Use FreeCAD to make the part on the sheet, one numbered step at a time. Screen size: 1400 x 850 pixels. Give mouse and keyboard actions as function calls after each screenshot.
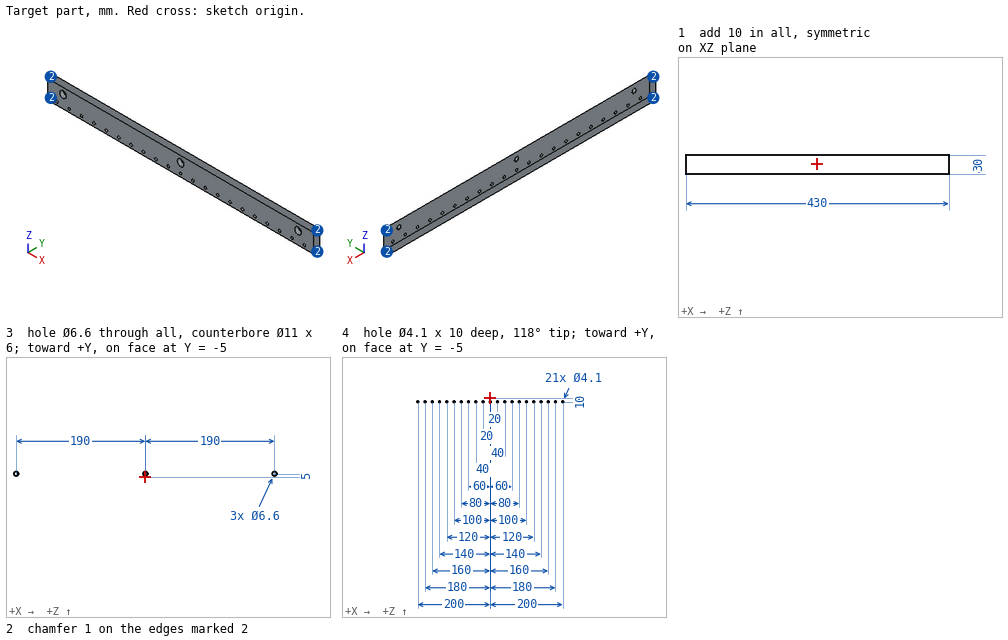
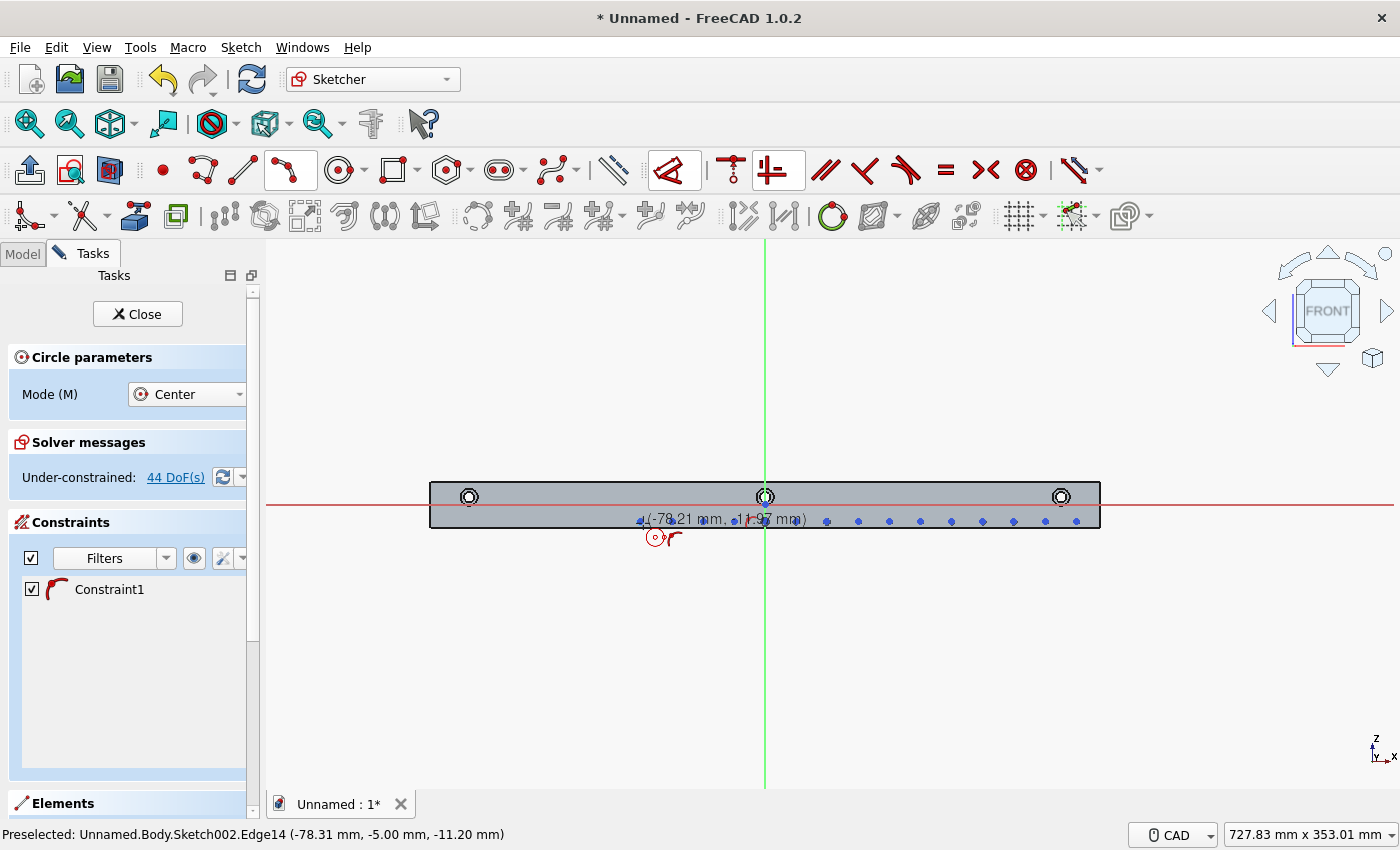
click(609, 521)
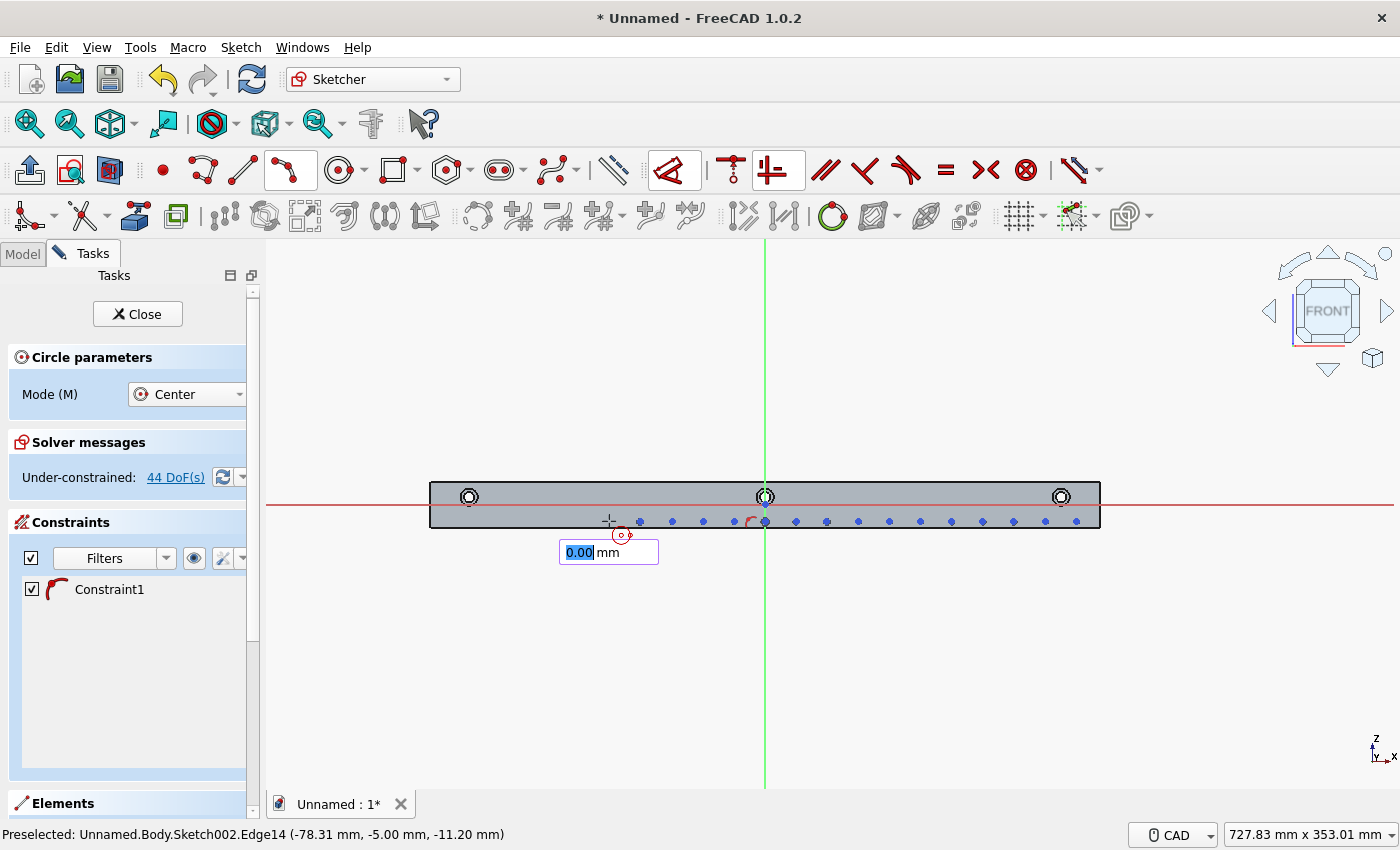
scroll(612, 523, up, 9)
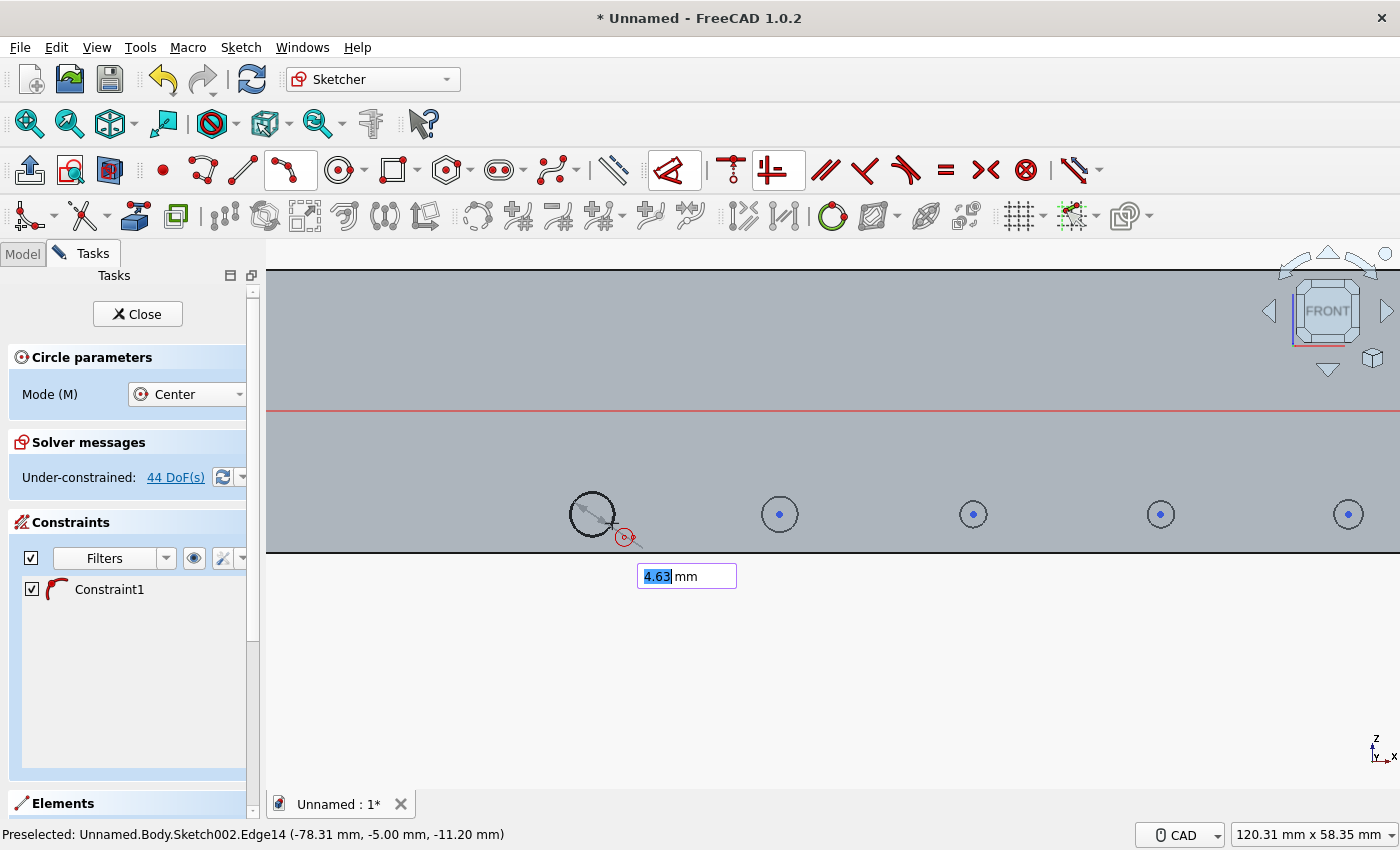
click(608, 519)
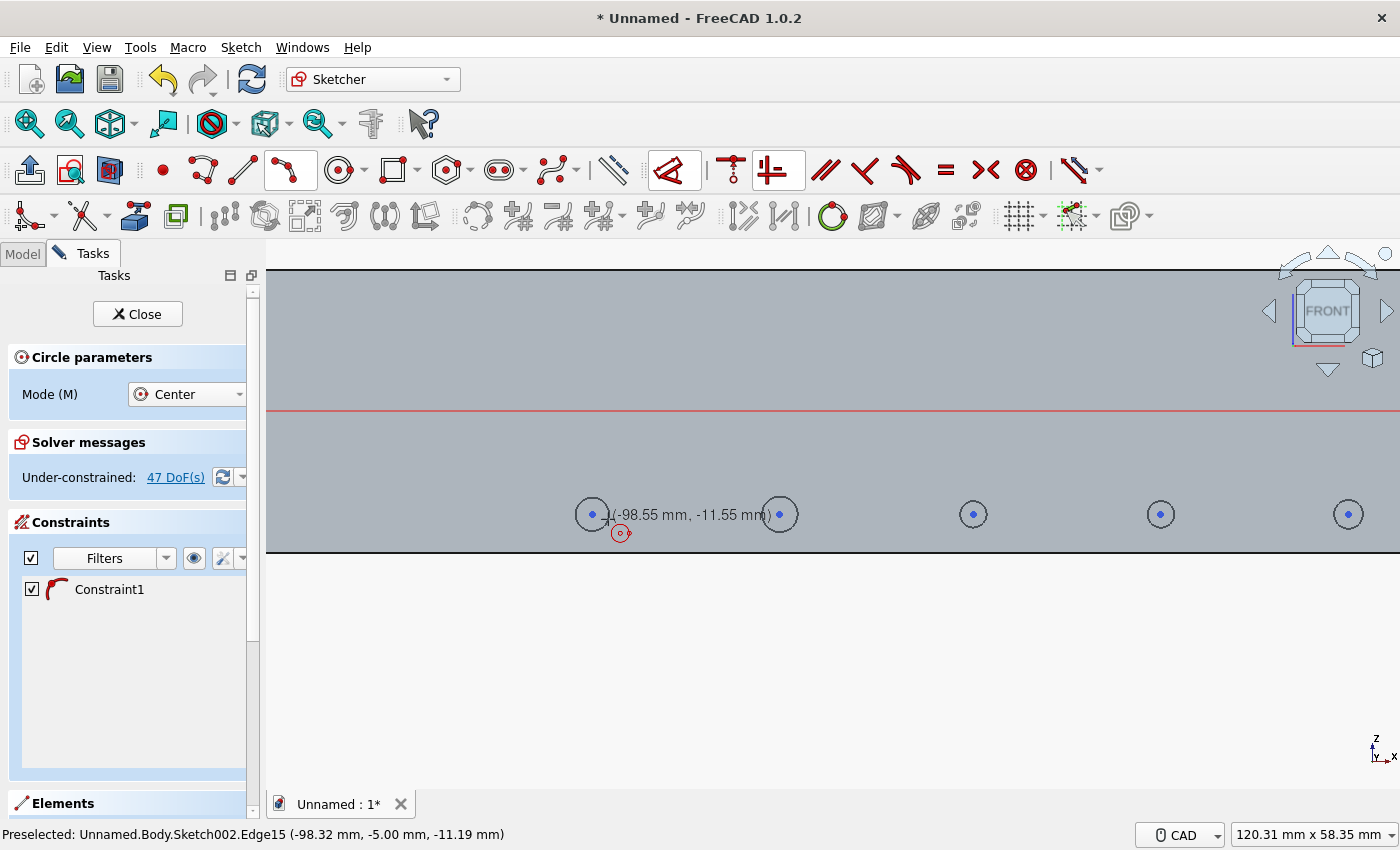
scroll(612, 523, down, 9)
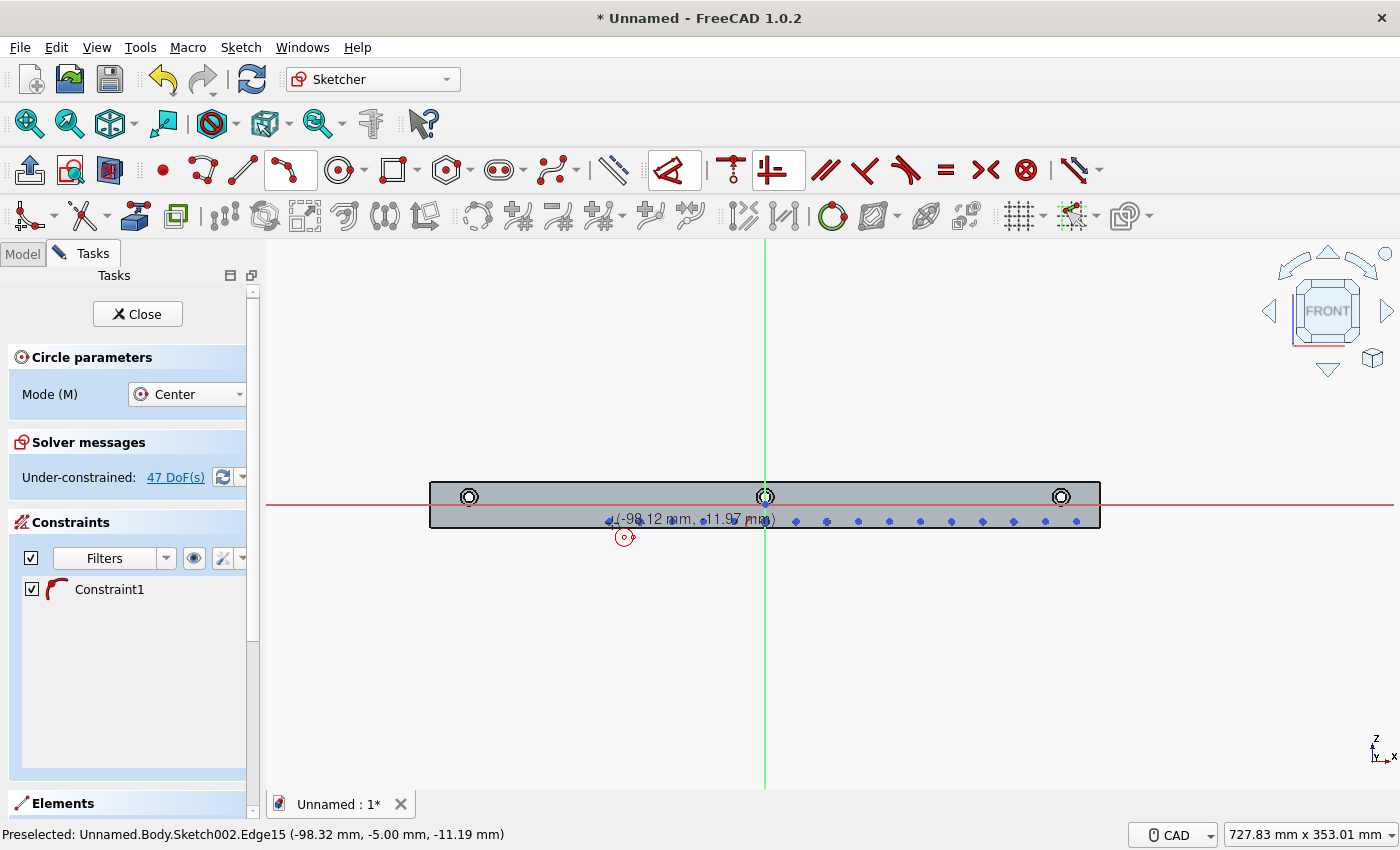
click(578, 521)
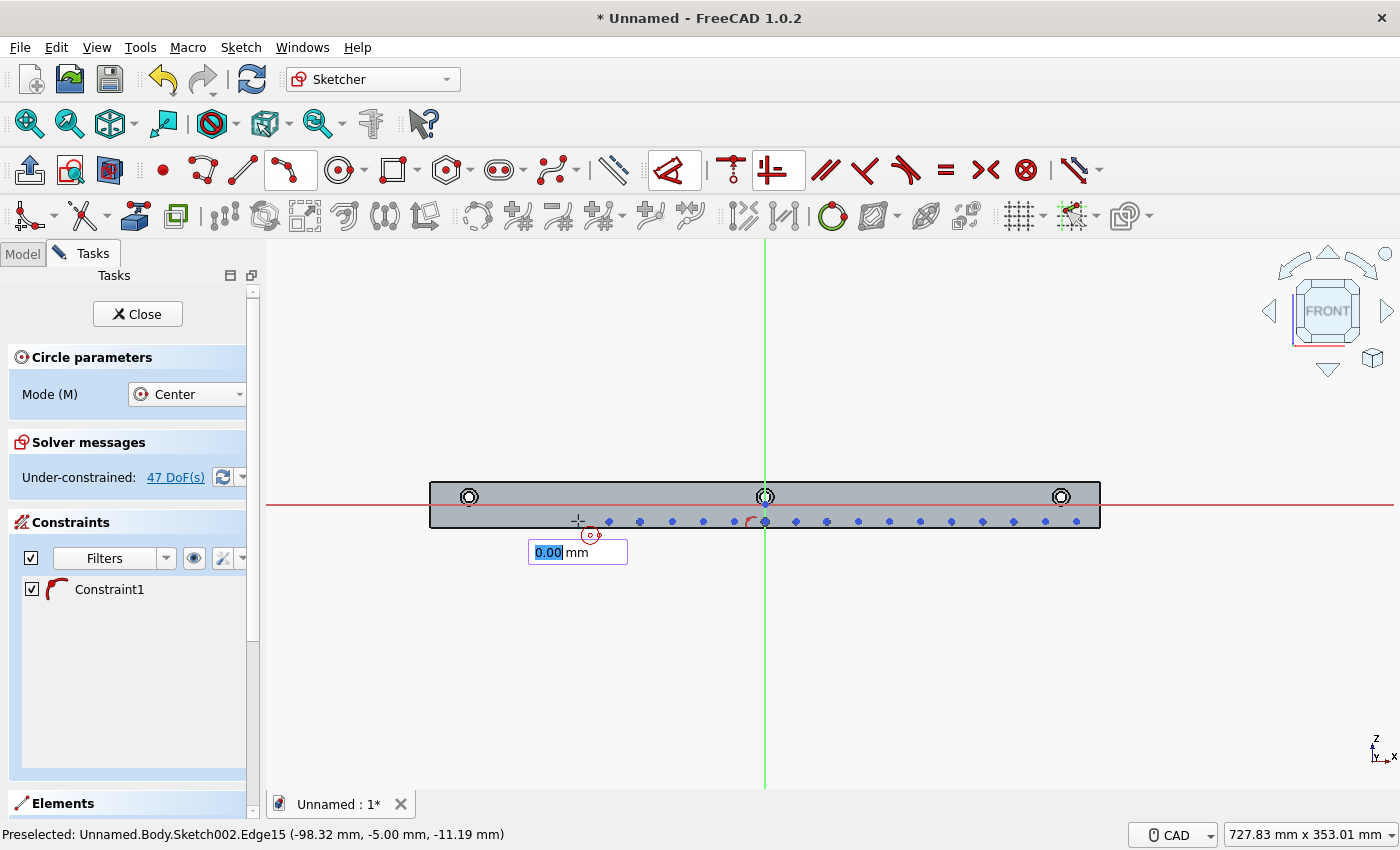
scroll(580, 523, up, 9)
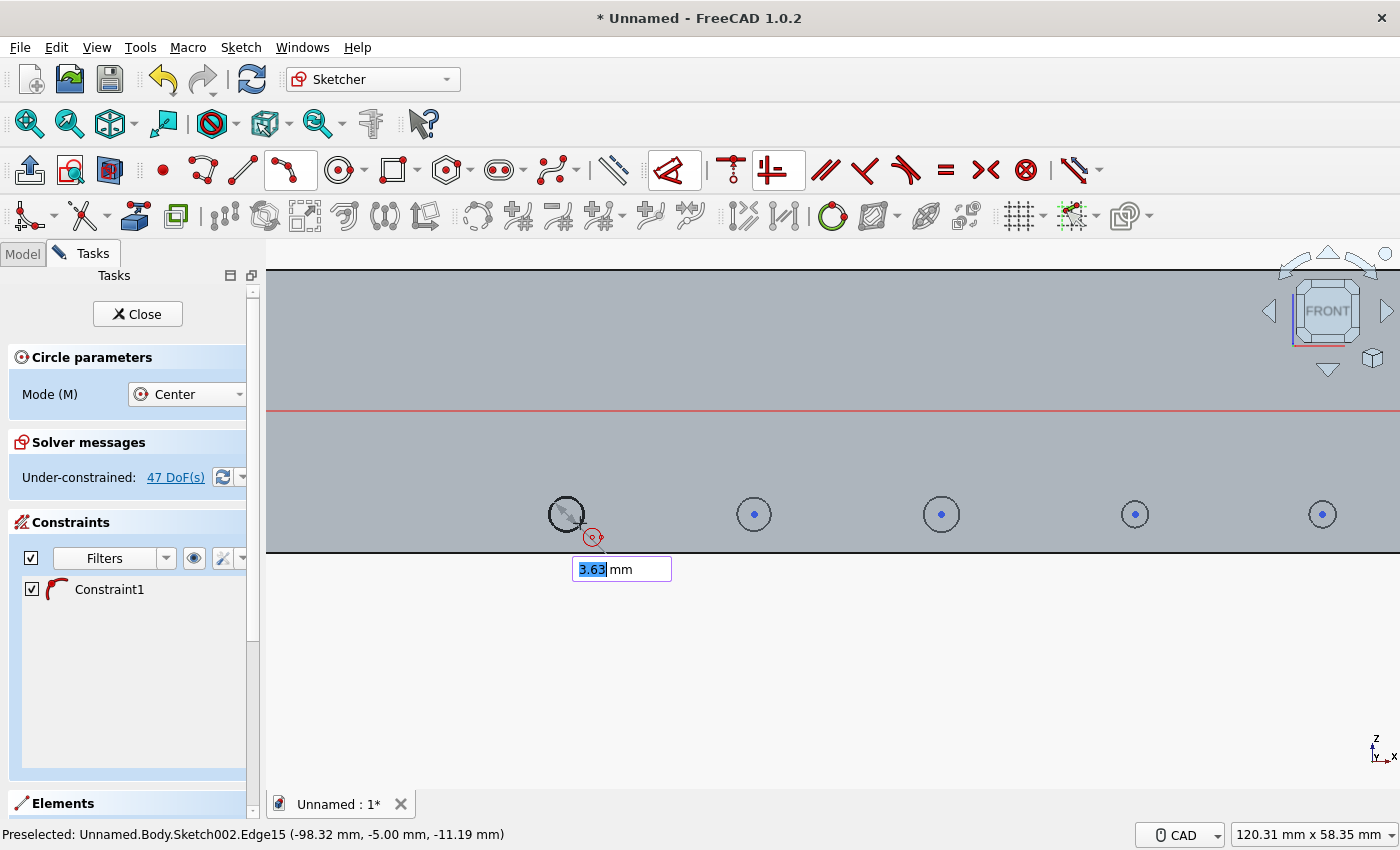
click(581, 519)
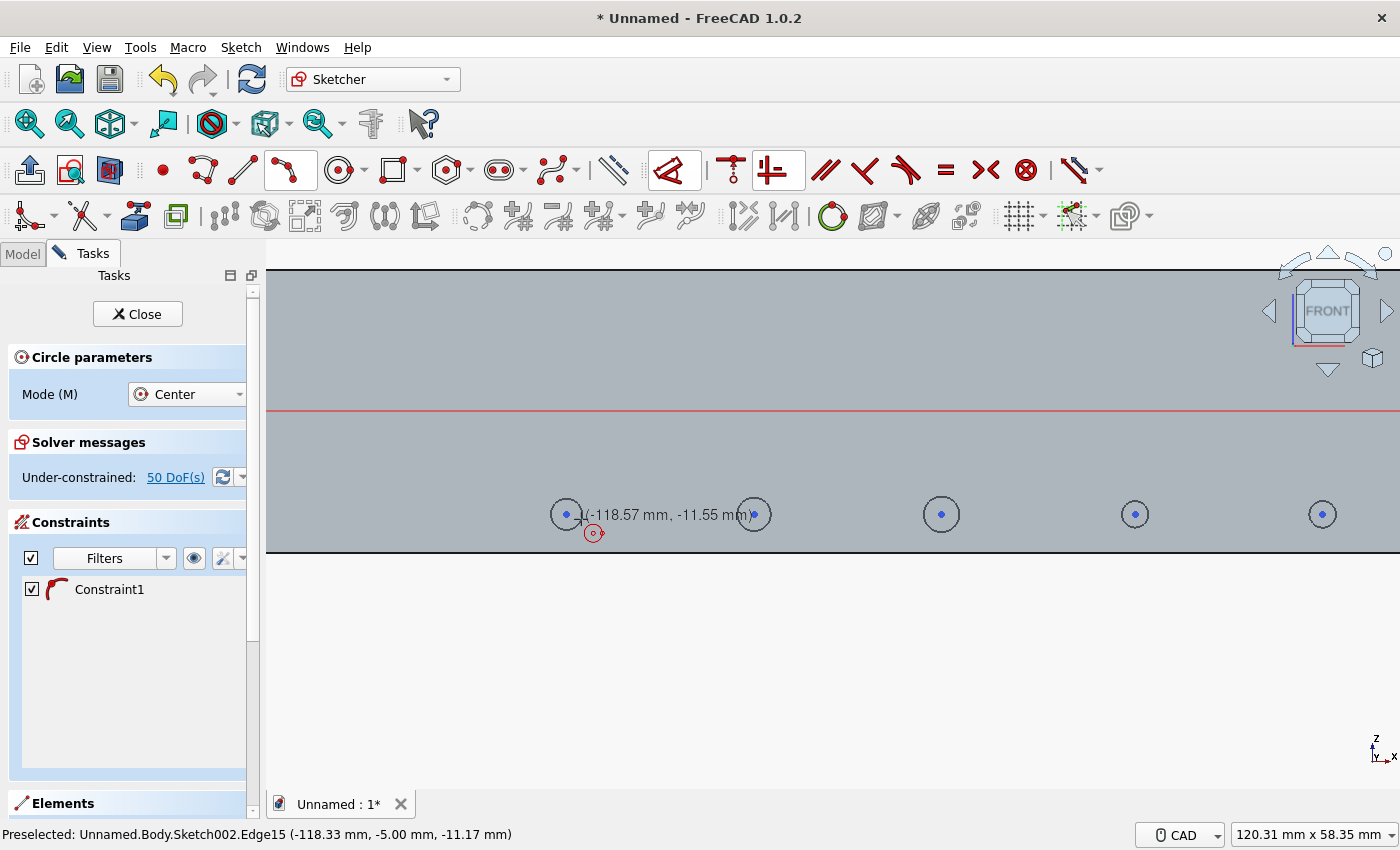
scroll(580, 523, down, 9)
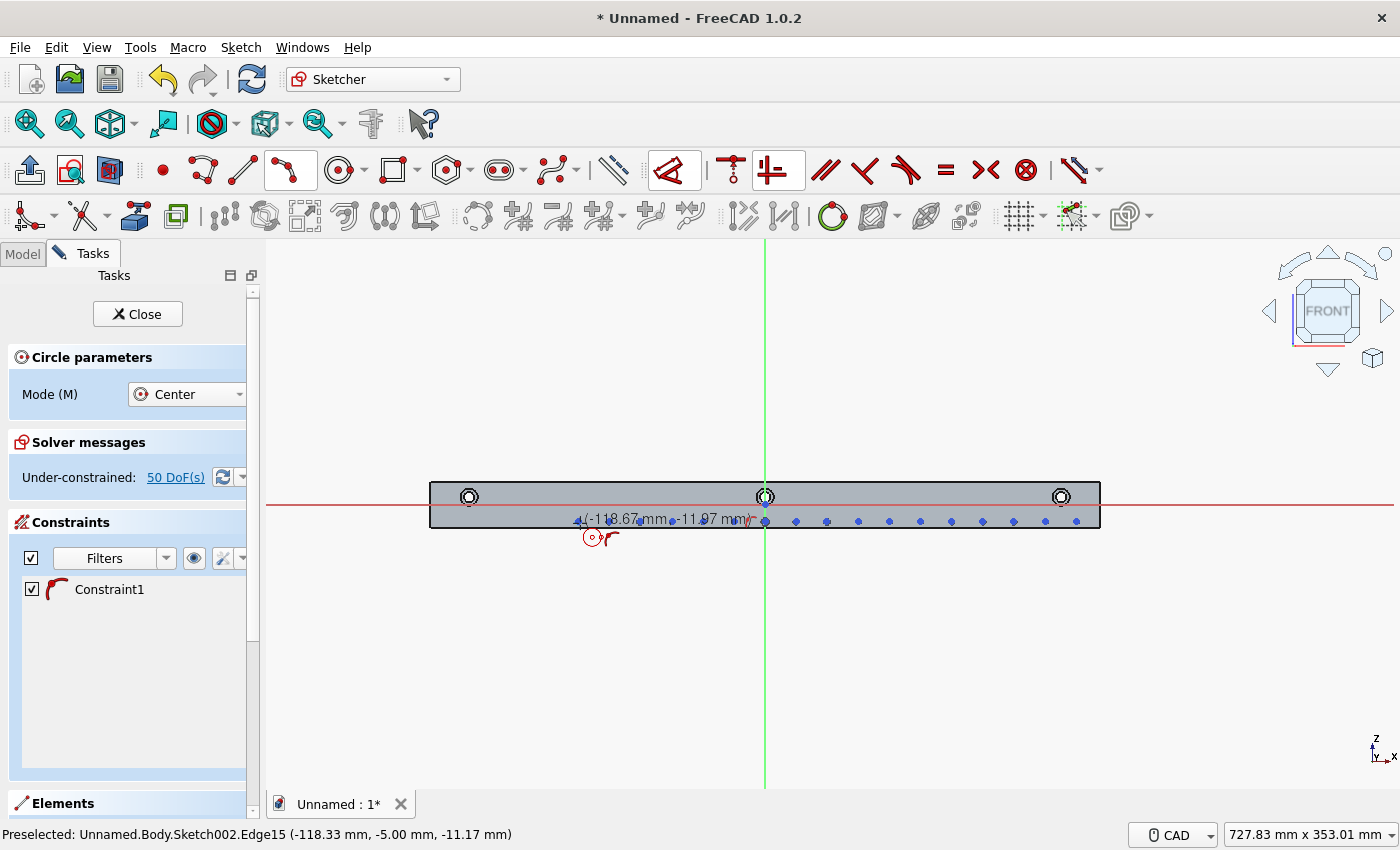
click(547, 521)